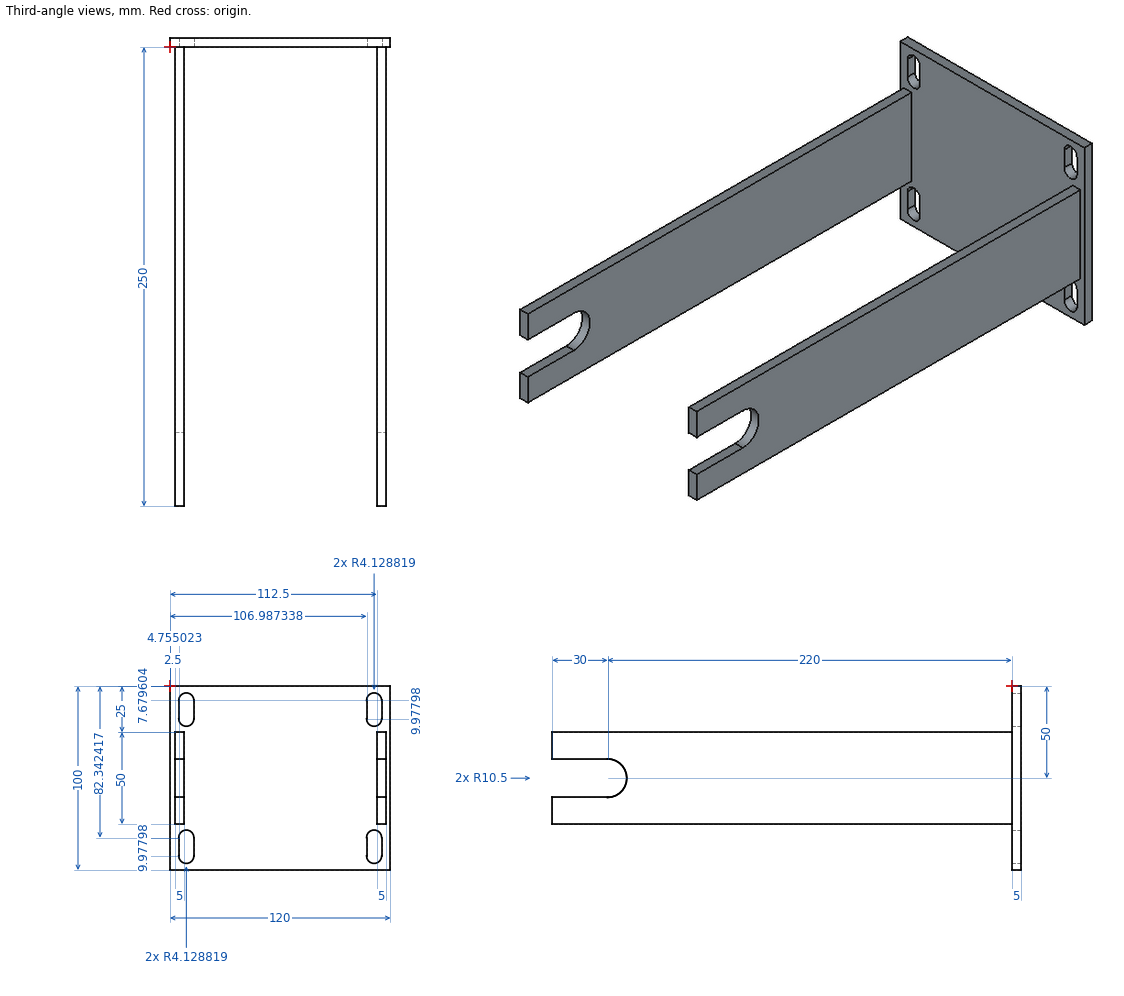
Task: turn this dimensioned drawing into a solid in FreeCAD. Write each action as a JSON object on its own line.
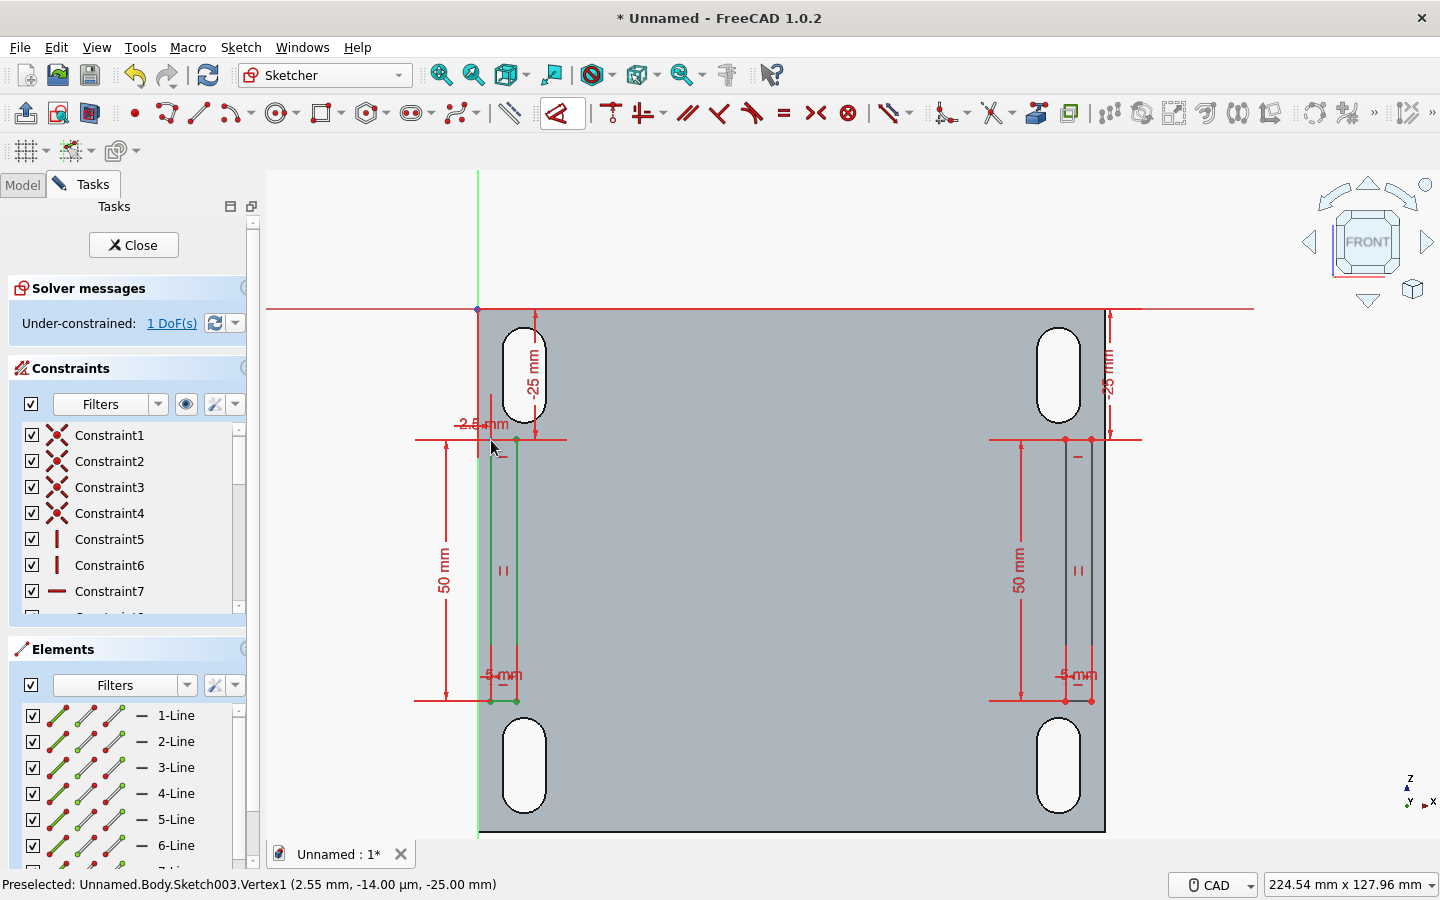
{"action": "left_click", "coordinate": [1066, 440]}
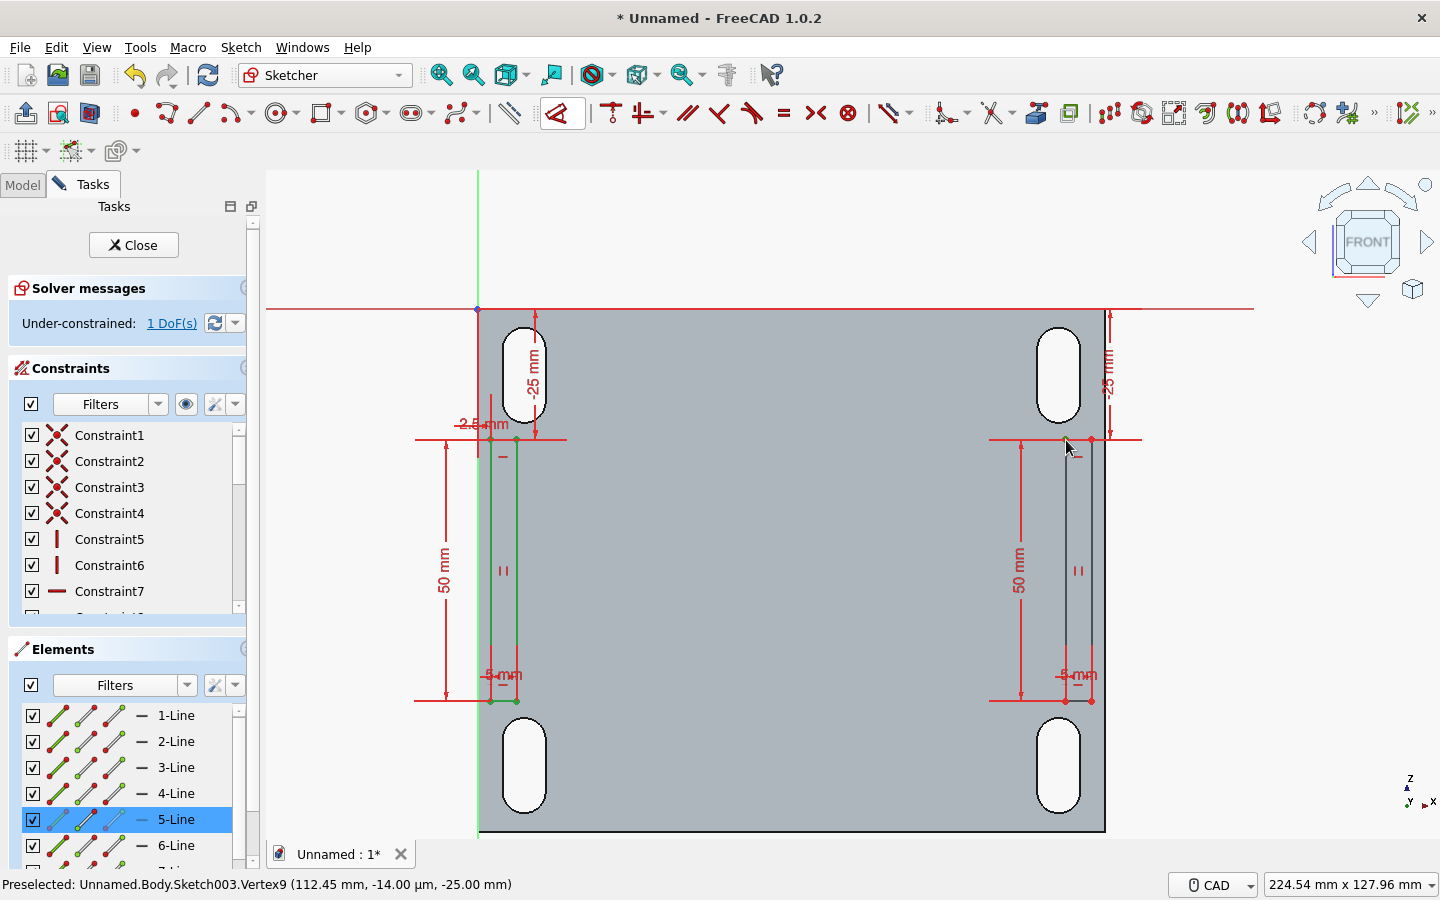
{"action": "left_click", "coordinate": [580, 114]}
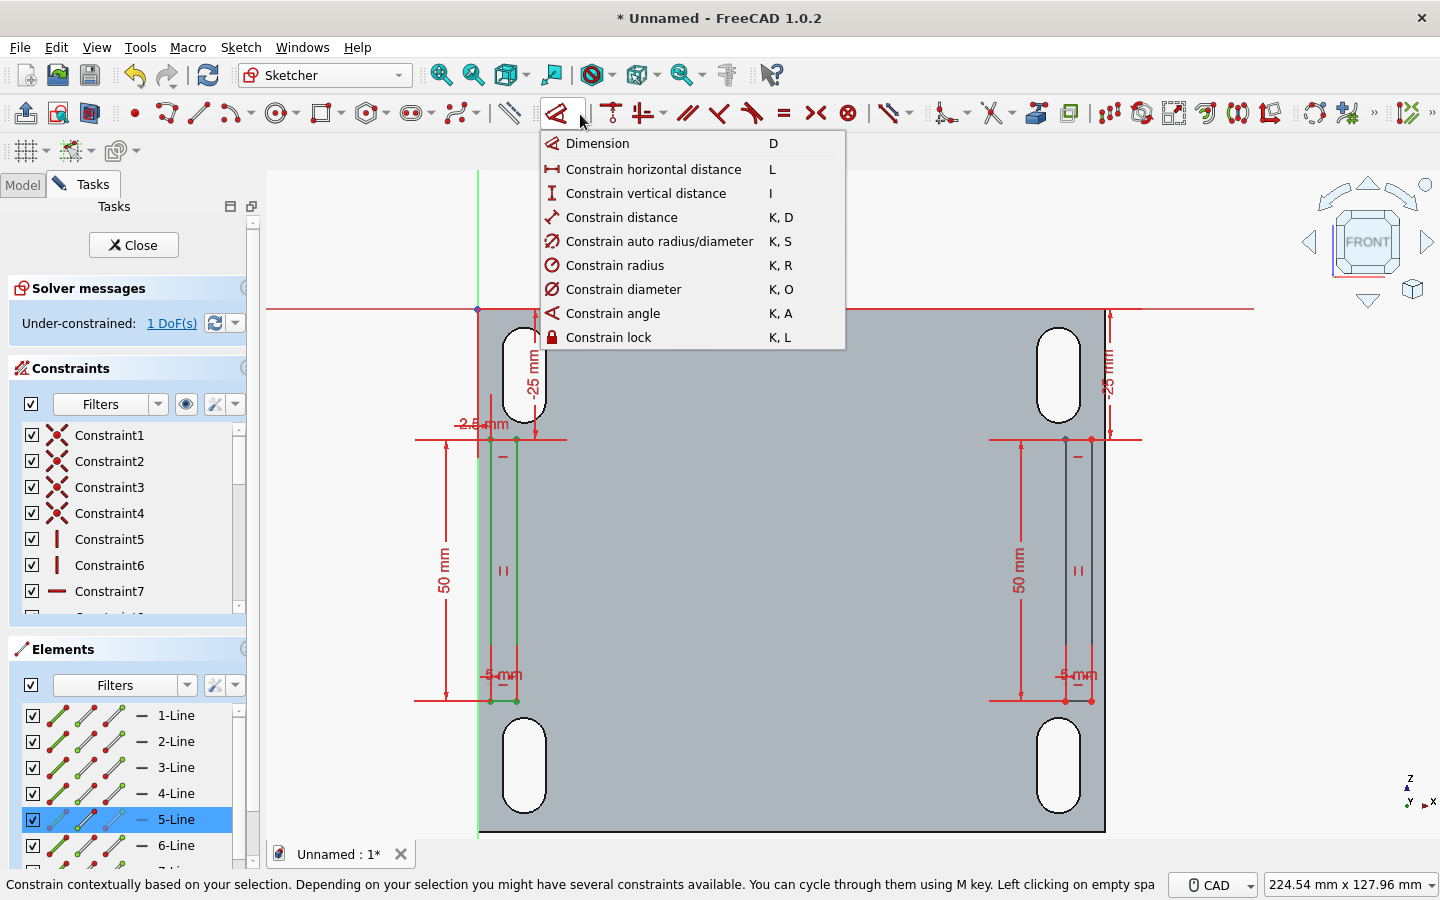
{"action": "left_click", "coordinate": [693, 169]}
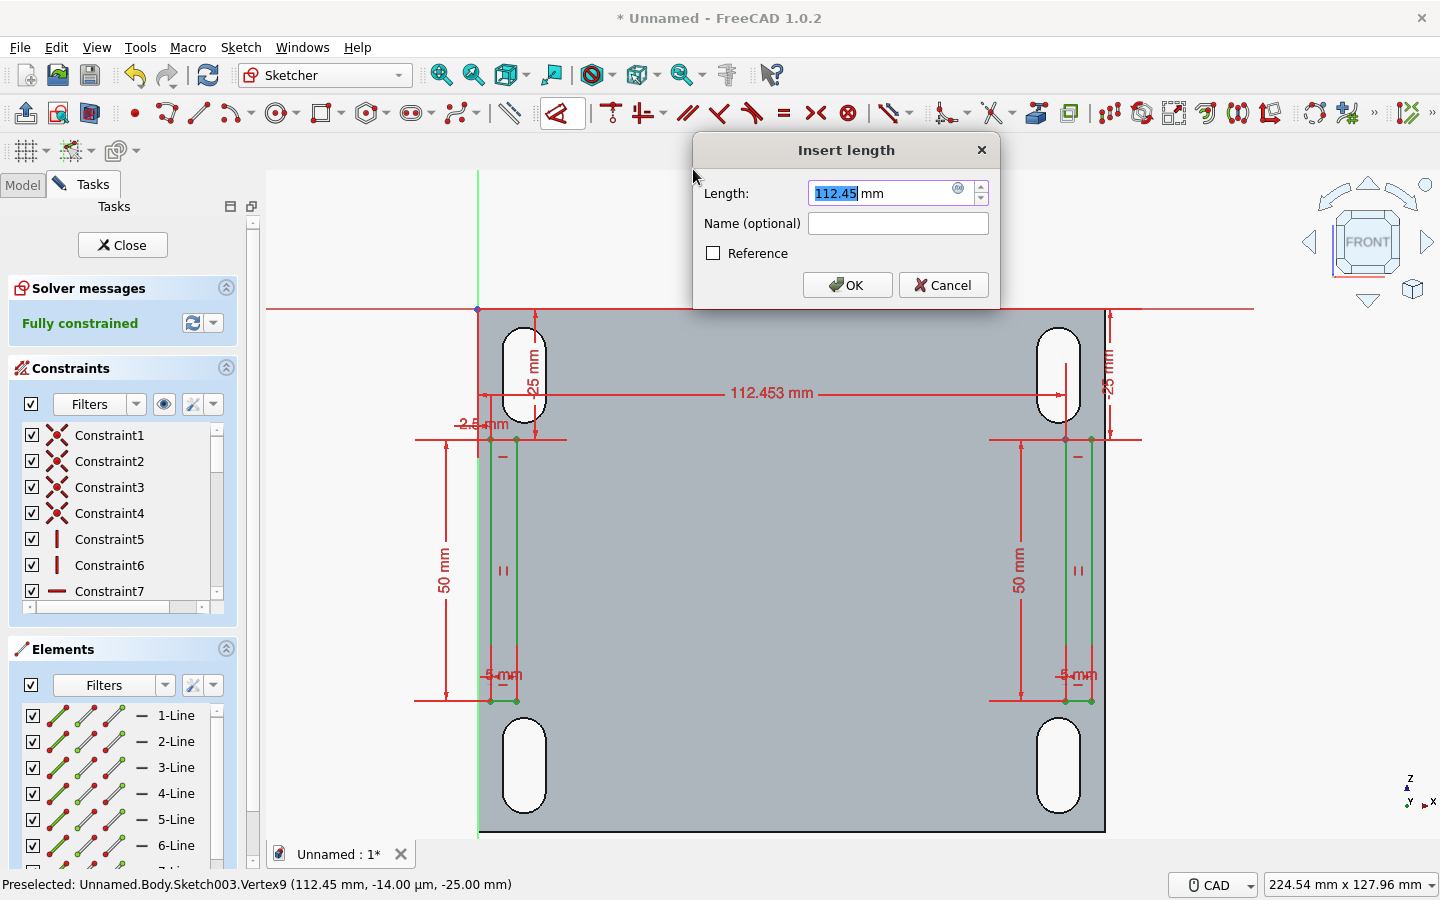
{"action": "type", "text": "112.5"}
{"action": "key", "text": "Return"}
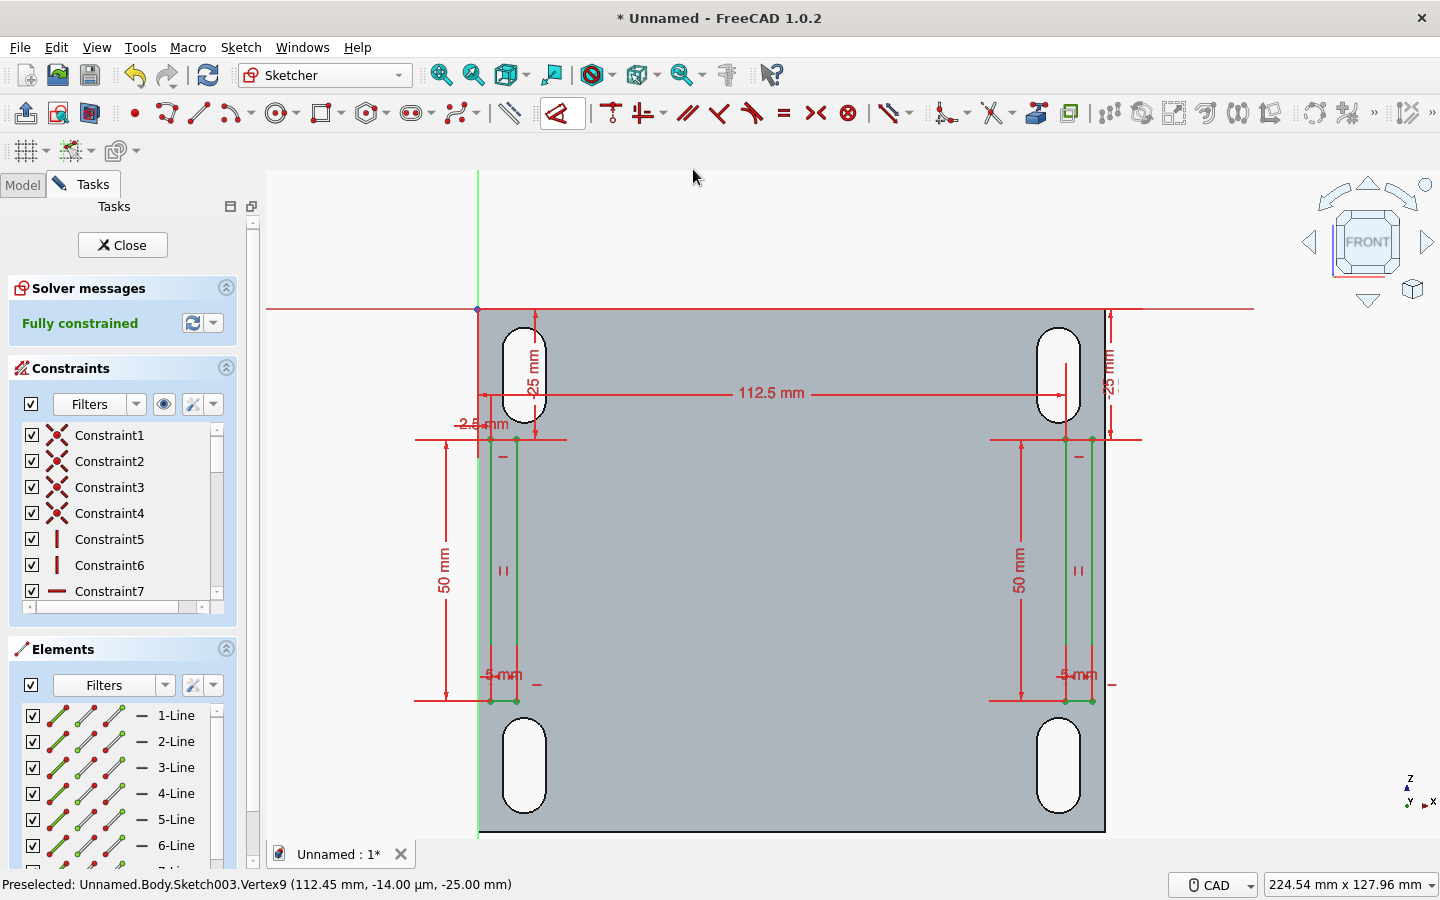
{"action": "left_click", "coordinate": [123, 245]}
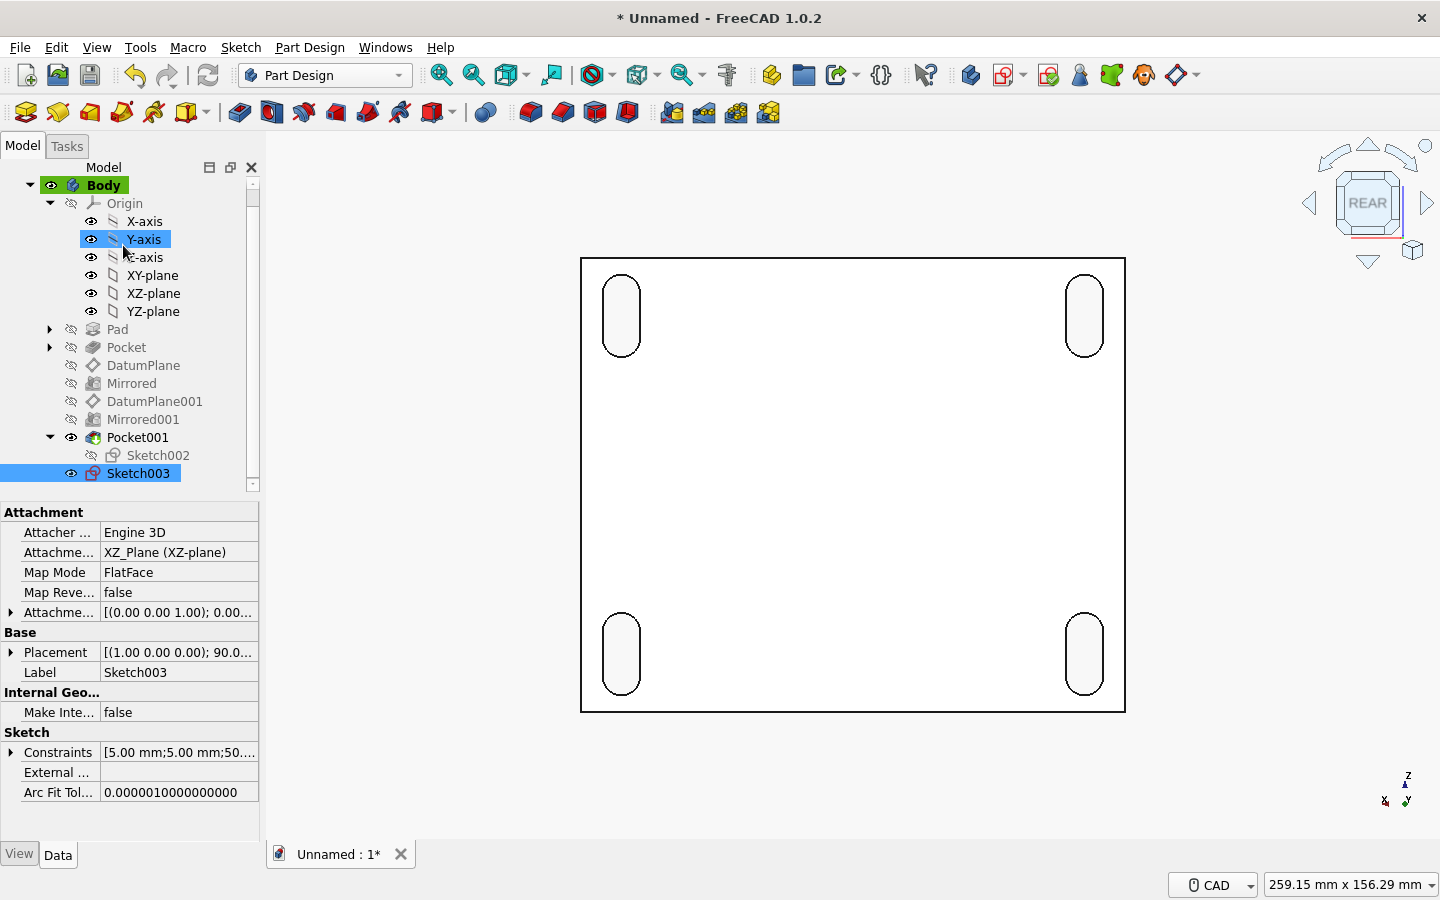
{"action": "left_click", "coordinate": [26, 112]}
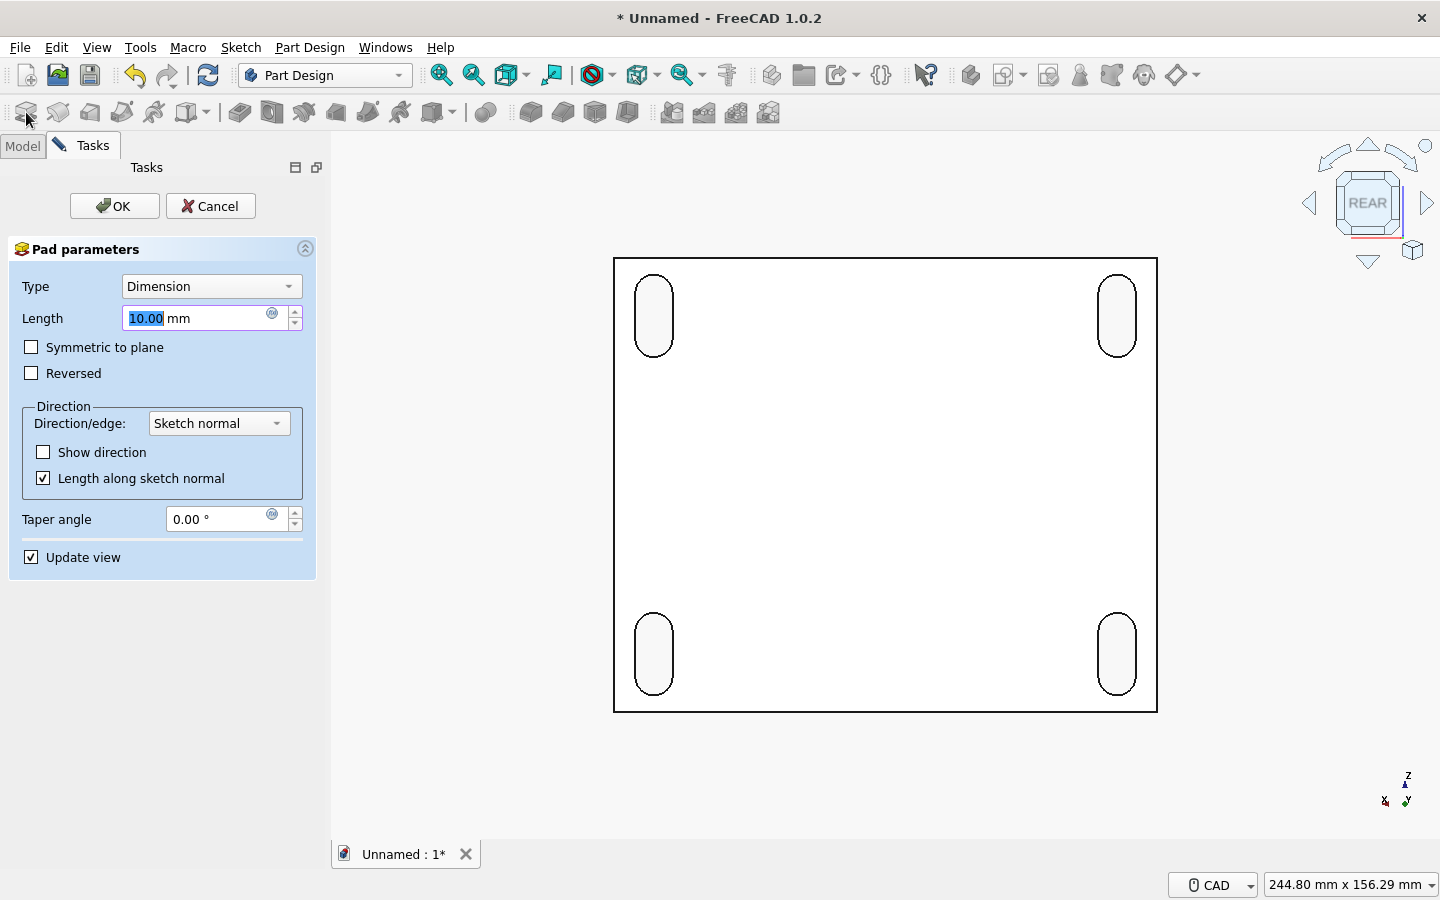
{"action": "type", "text": "250"}
{"action": "key", "text": "Tab"}